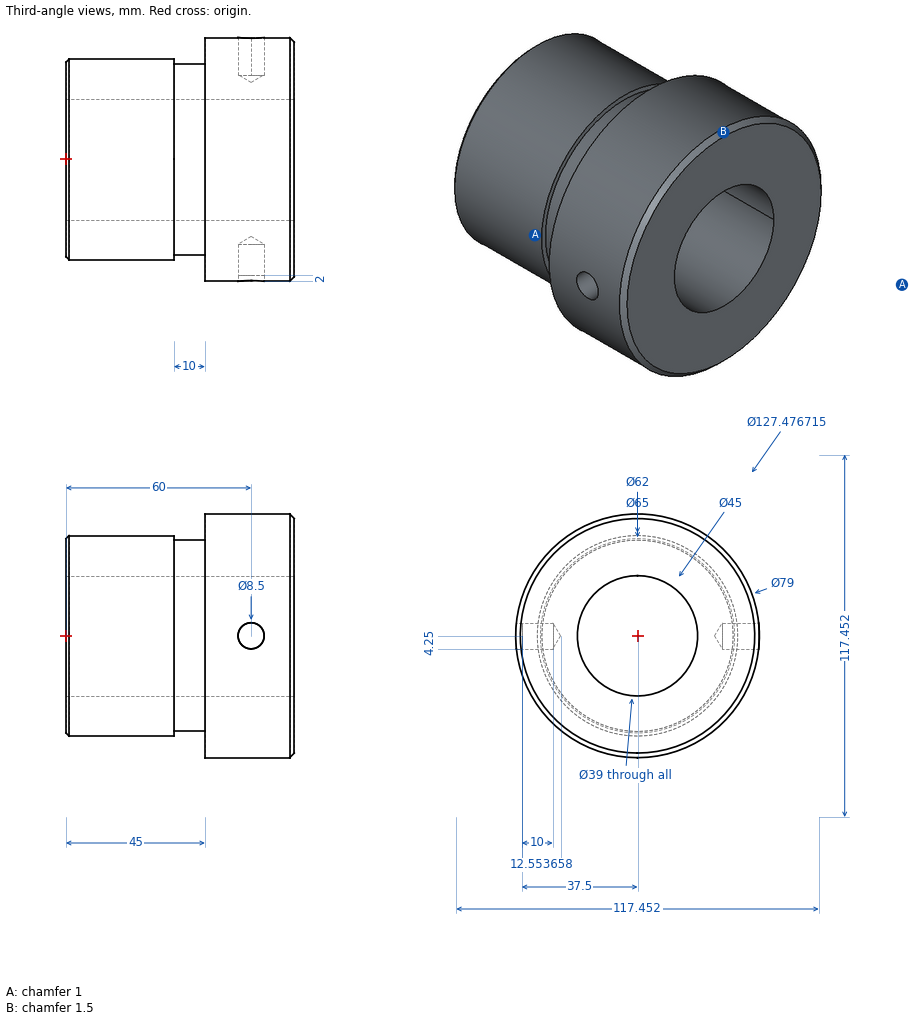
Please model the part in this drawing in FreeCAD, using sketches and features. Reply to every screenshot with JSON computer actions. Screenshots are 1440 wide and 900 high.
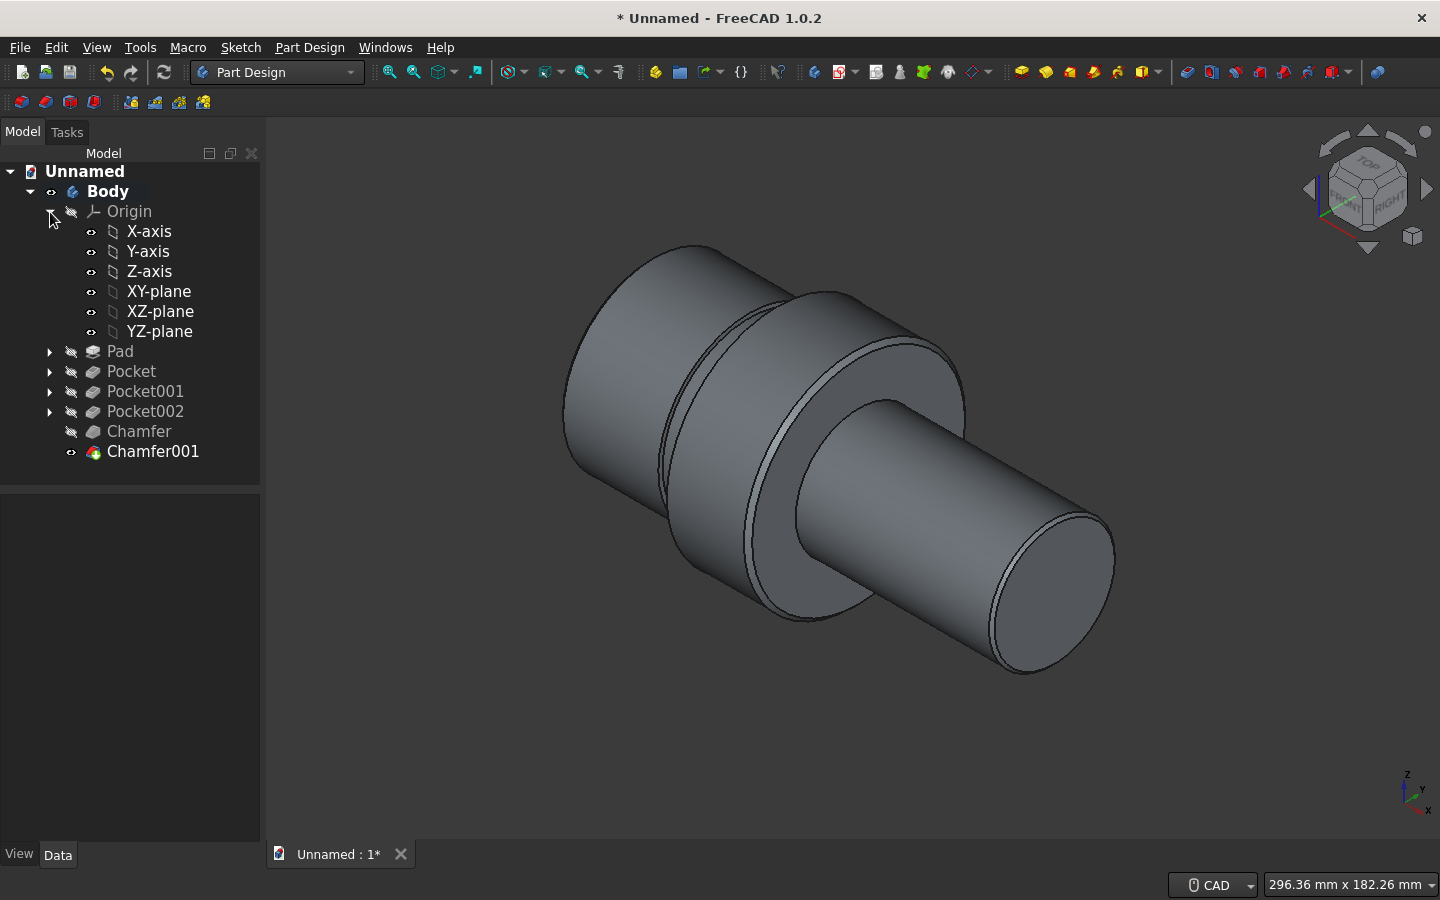
{"action": "left_click", "coordinate": [136, 312]}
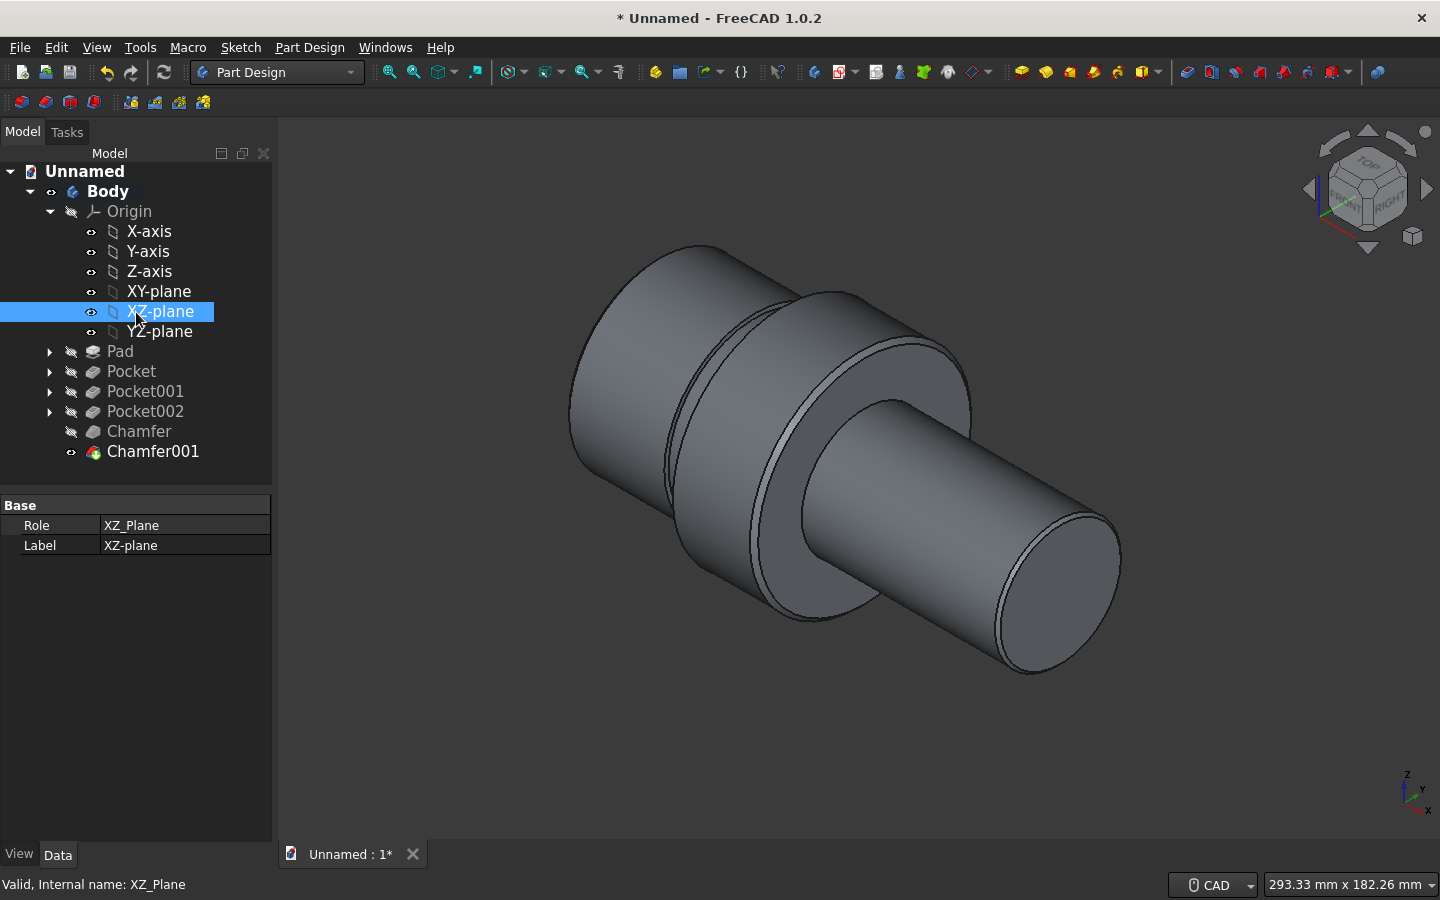
{"action": "left_click", "coordinate": [972, 72]}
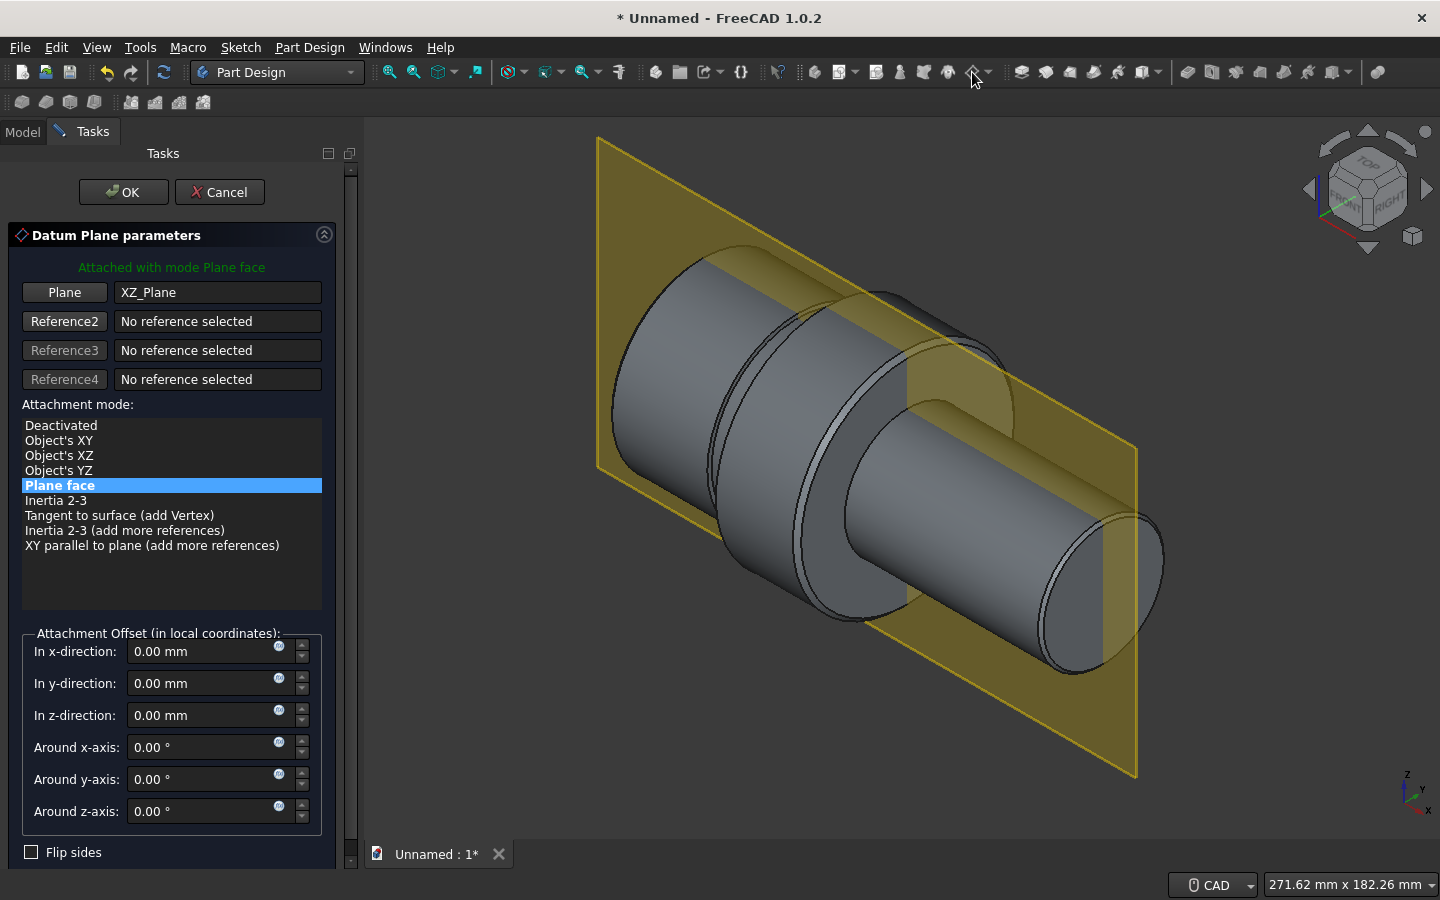
{"action": "triple_click", "coordinate": [210, 715]}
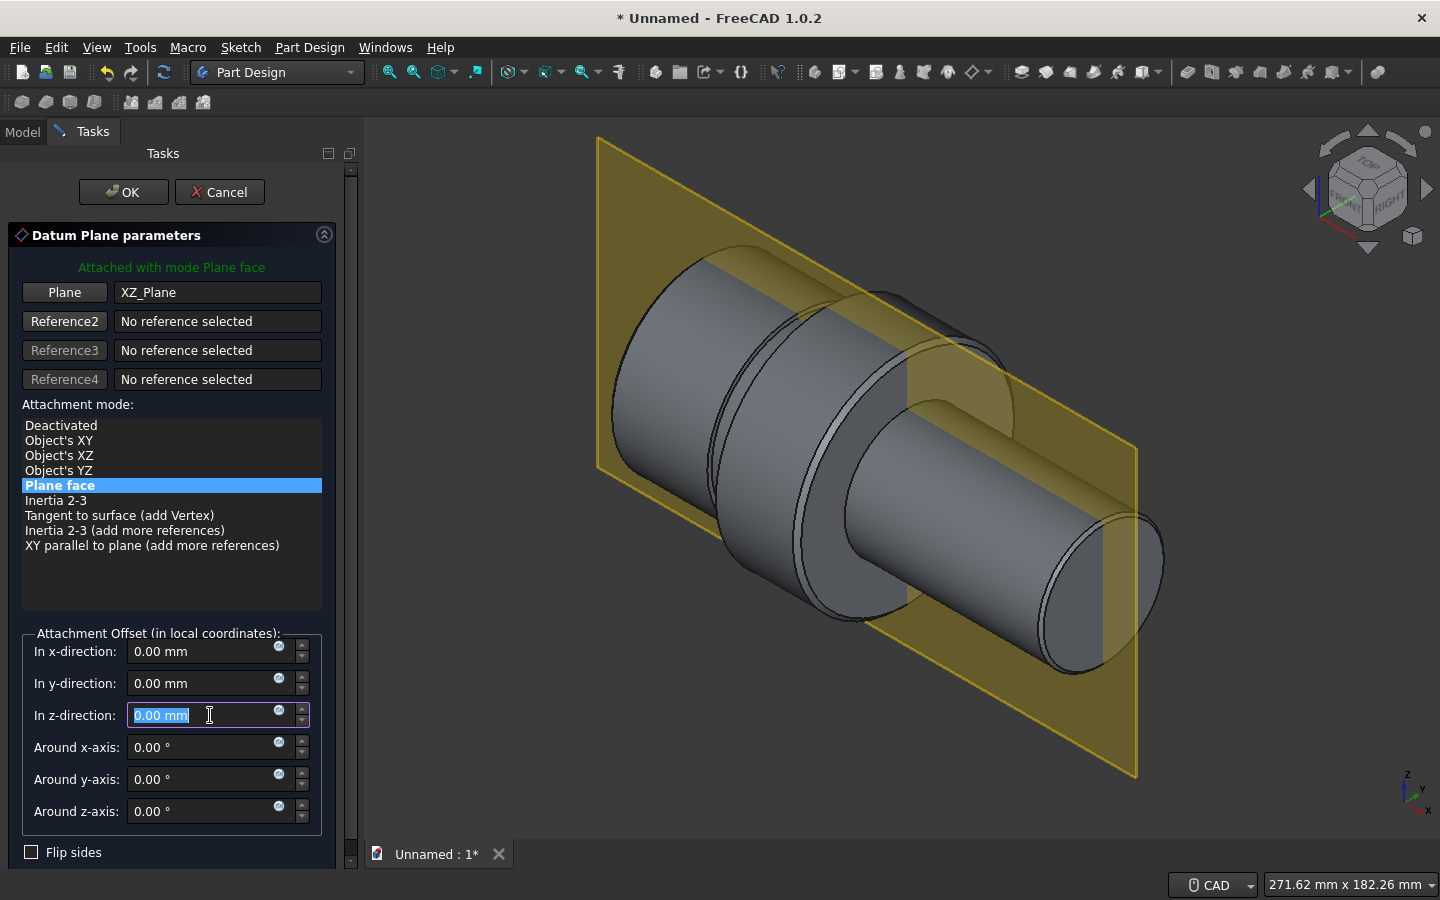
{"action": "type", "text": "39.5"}
{"action": "key", "text": "Tab"}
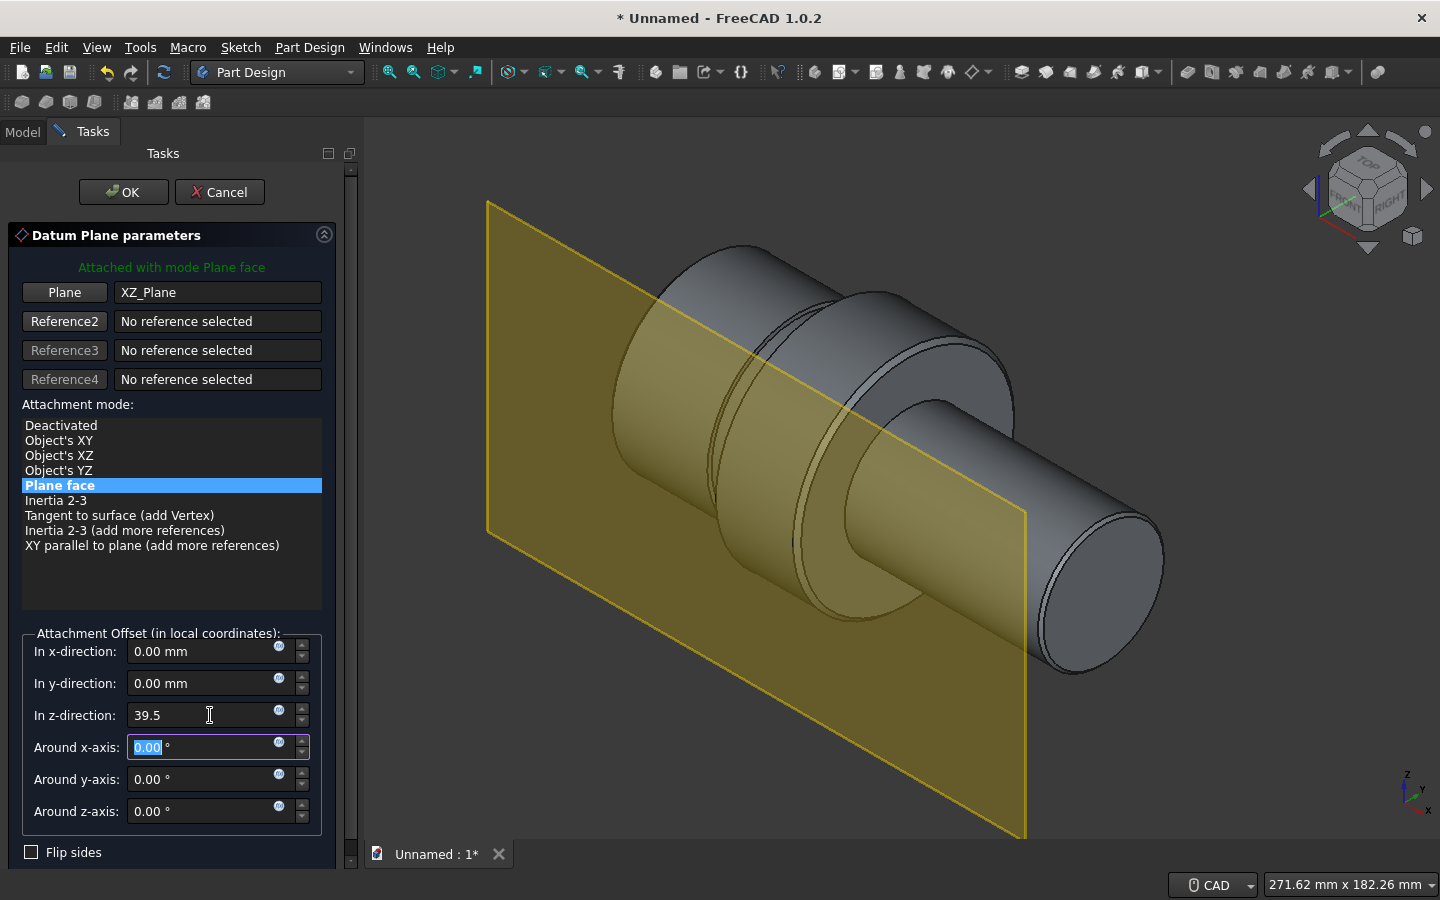
{"action": "left_click", "coordinate": [124, 192]}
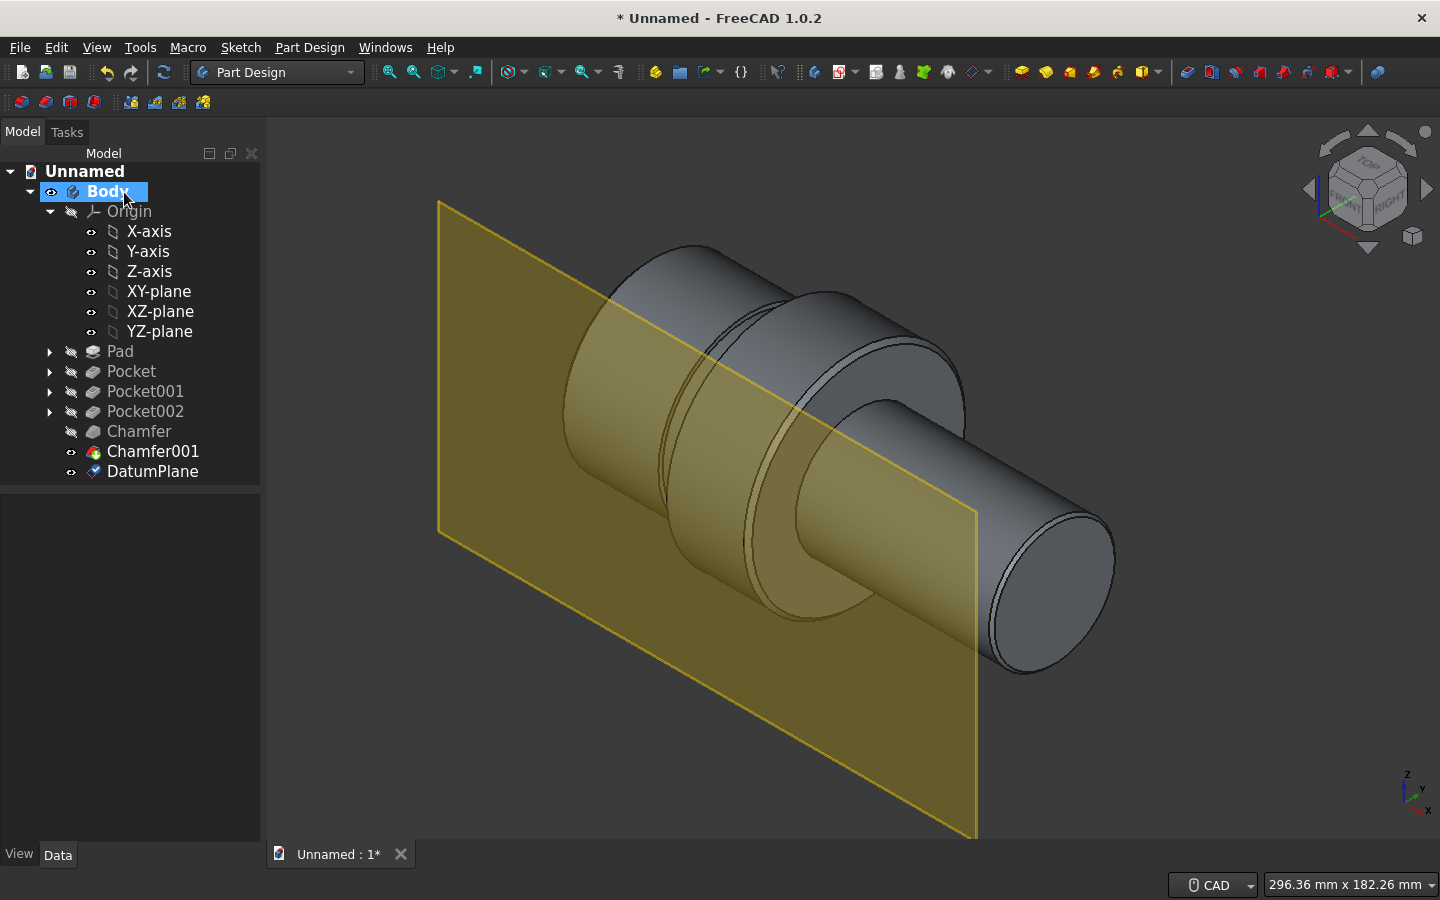
{"action": "left_click", "coordinate": [116, 472]}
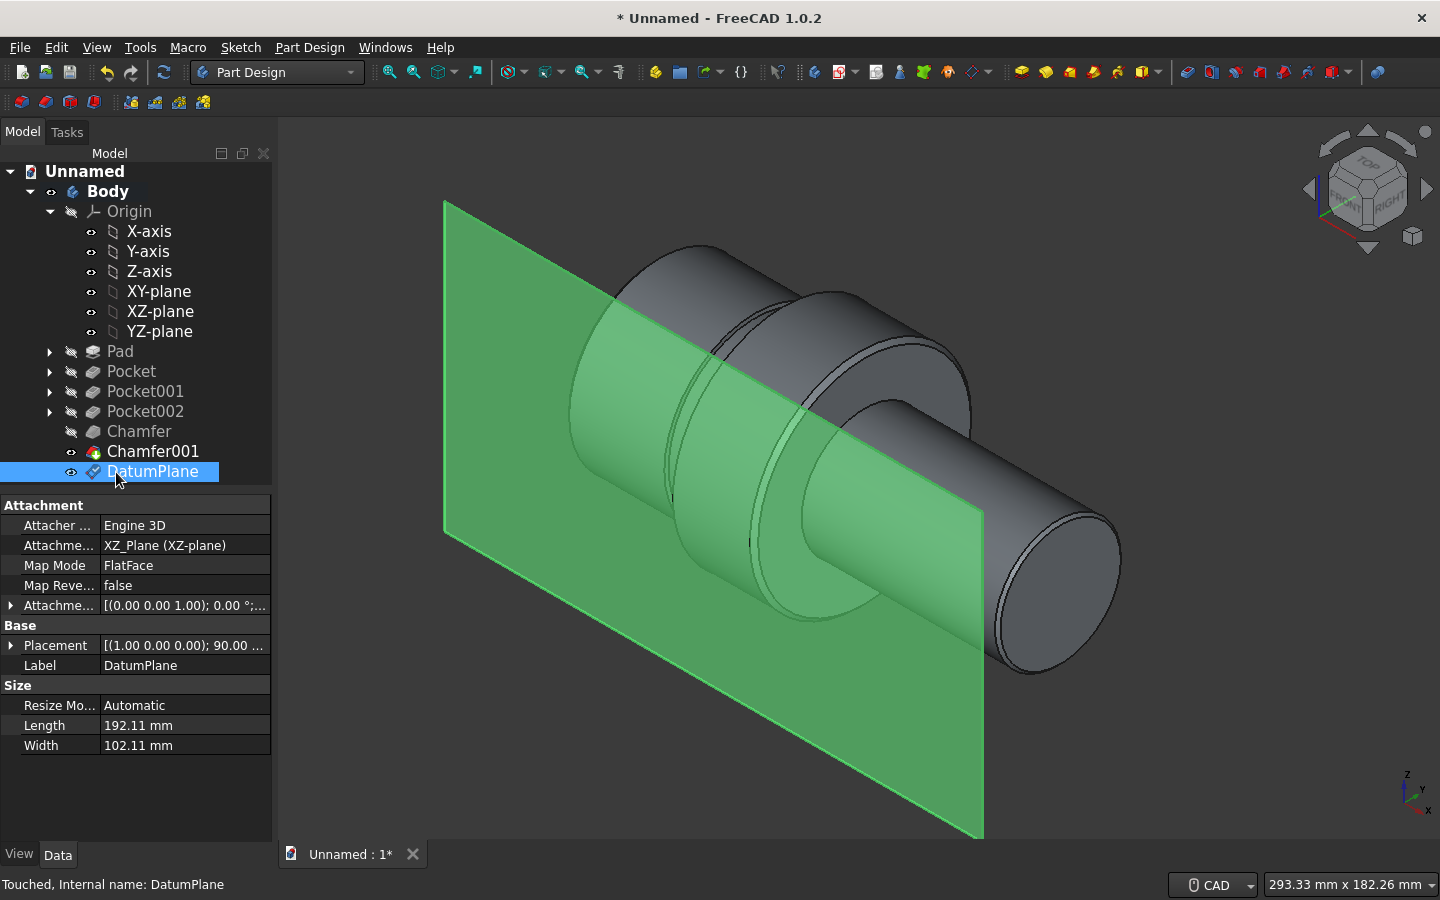
{"action": "left_click", "coordinate": [840, 72]}